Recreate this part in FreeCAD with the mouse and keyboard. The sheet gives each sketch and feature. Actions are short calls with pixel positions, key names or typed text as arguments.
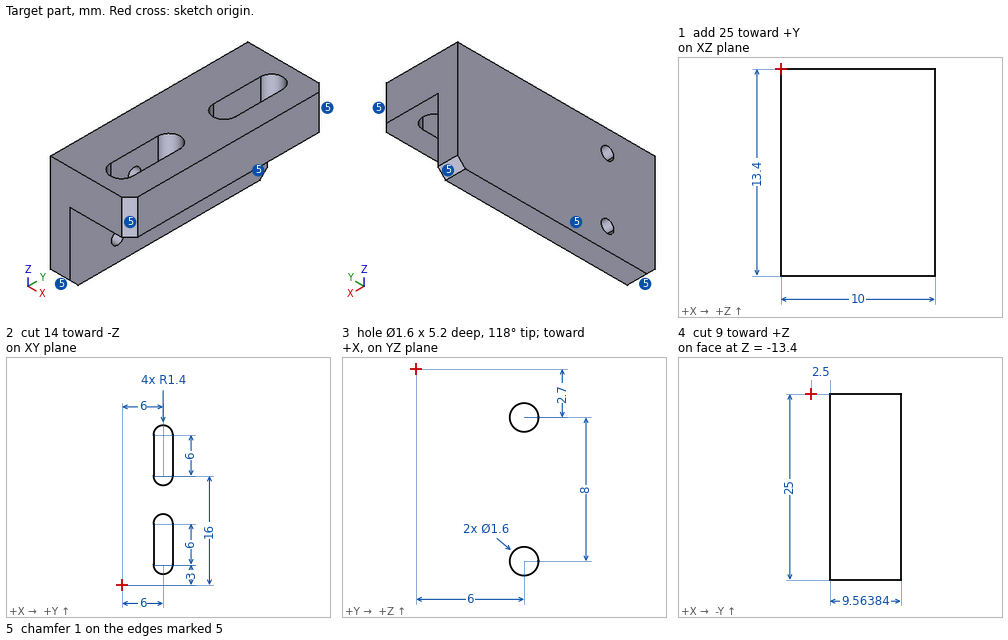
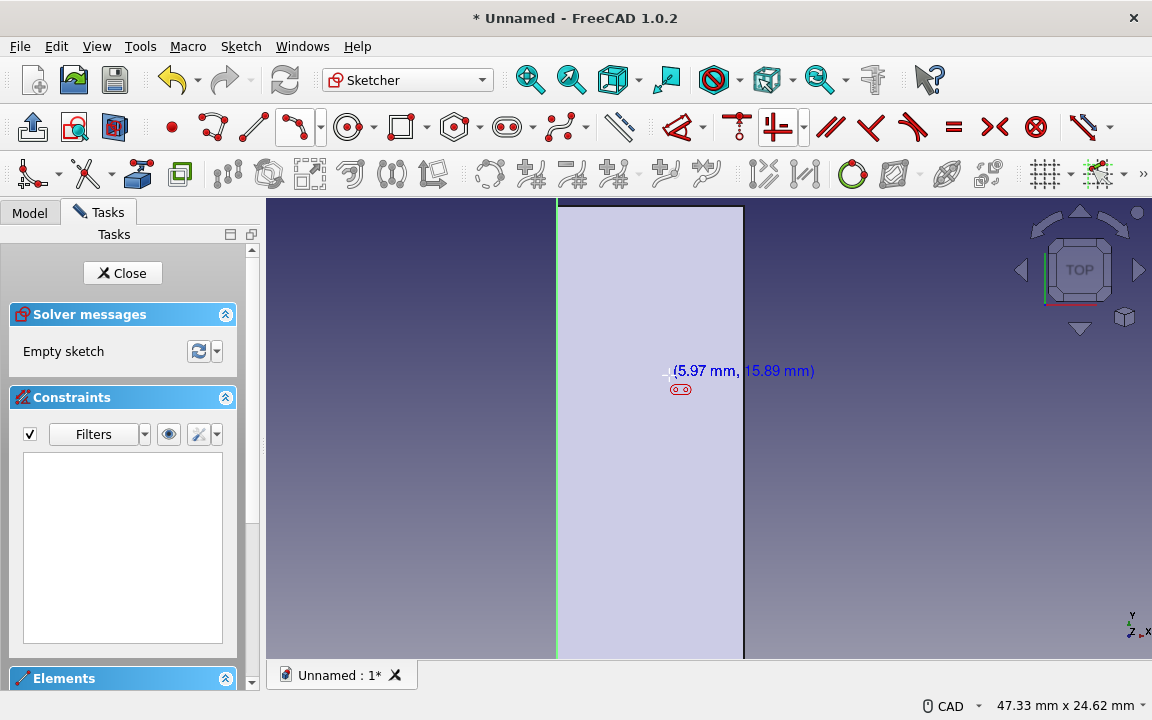
click(669, 374)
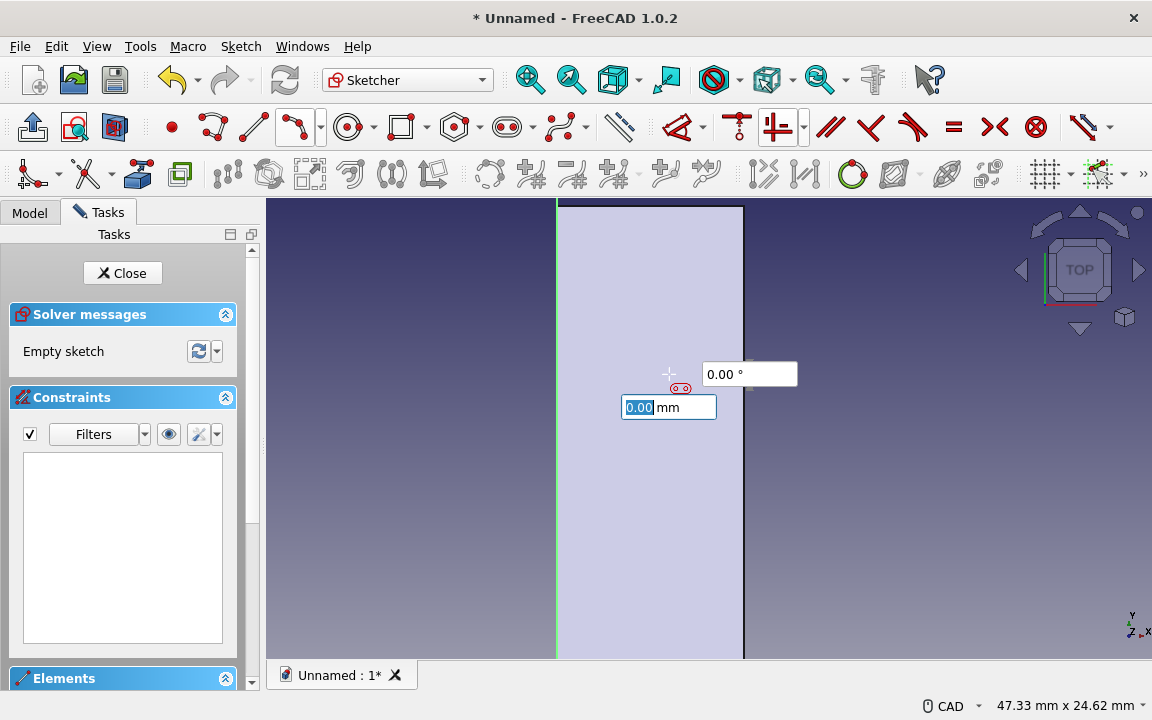
click(669, 262)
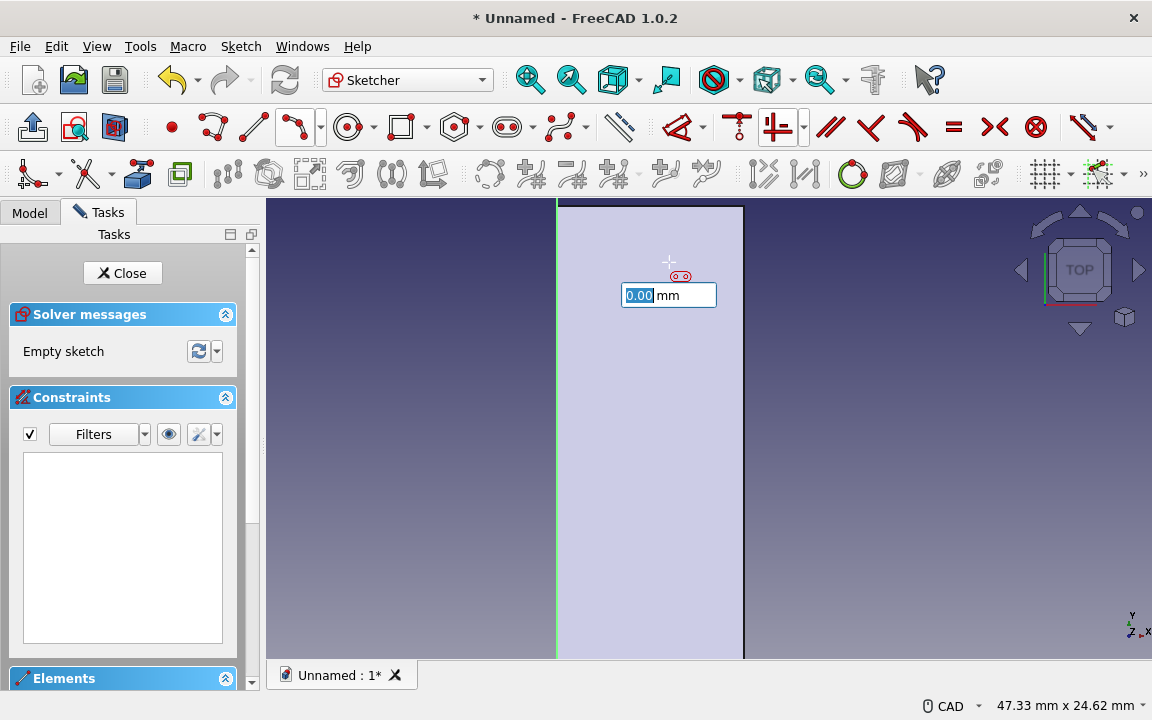
click(696, 318)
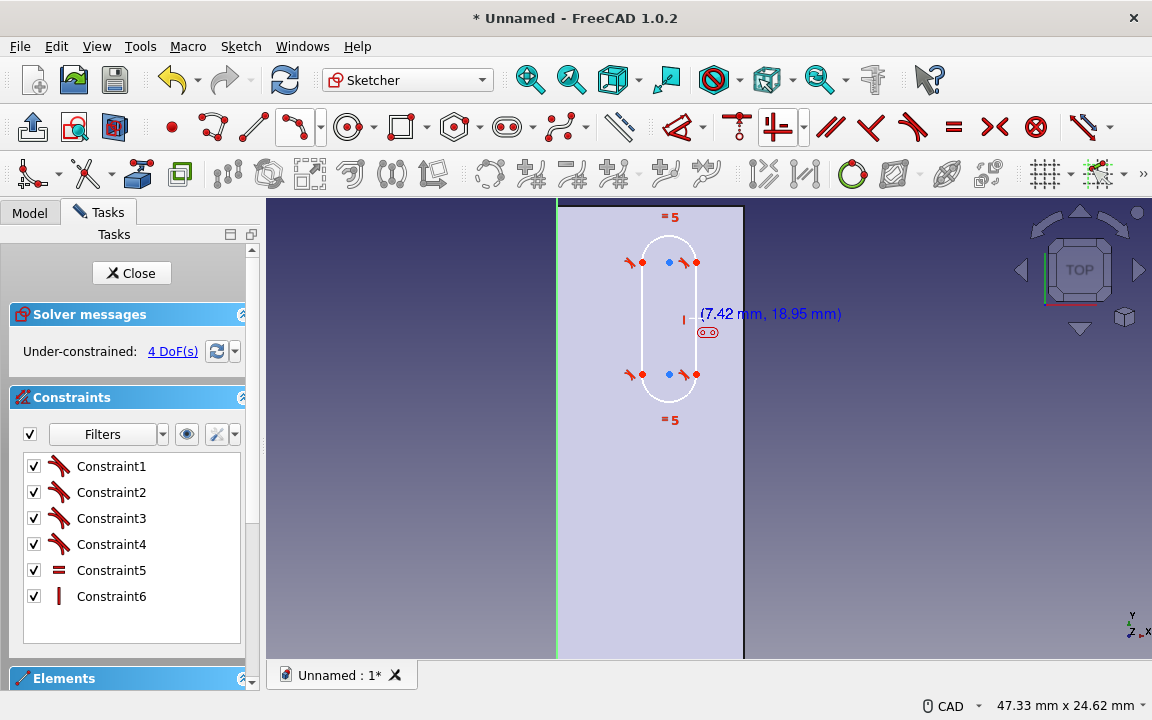
click(669, 618)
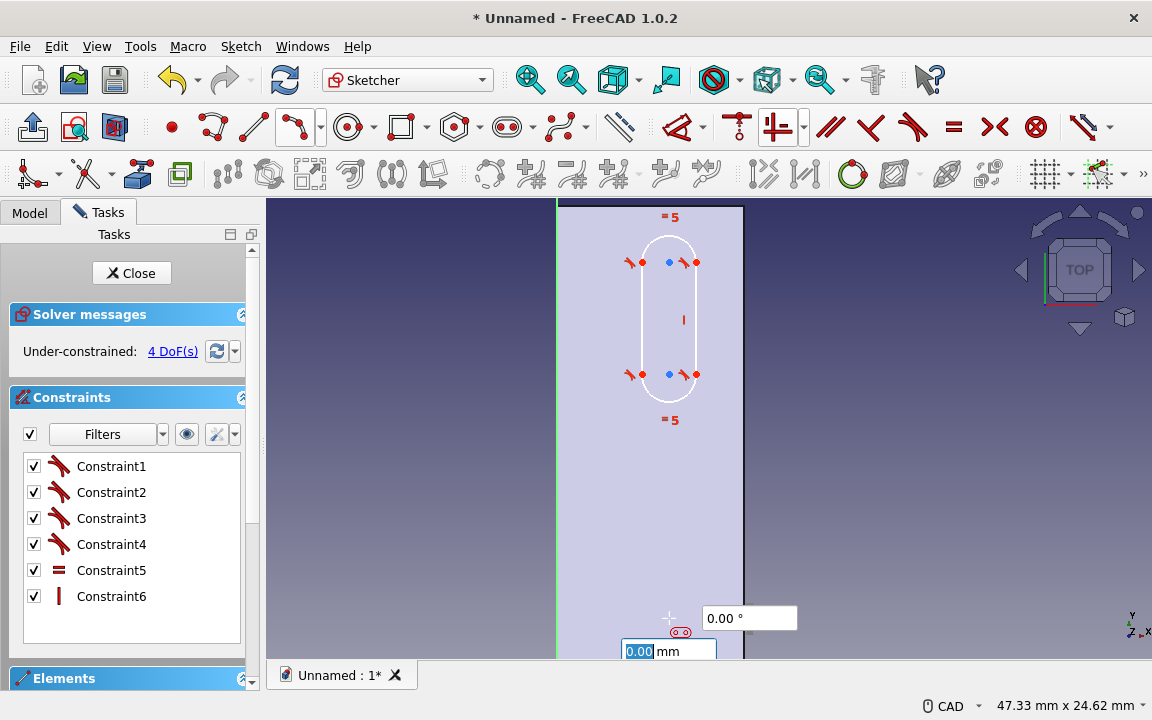
click(669, 505)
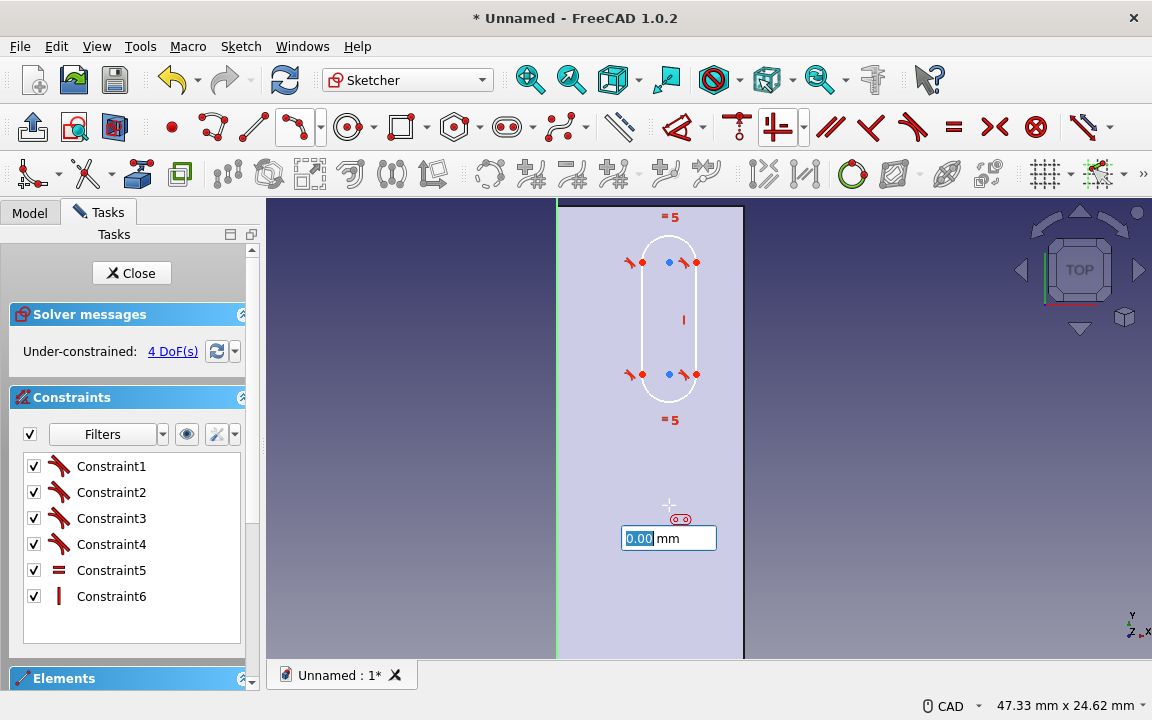
click(696, 561)
key(Escape)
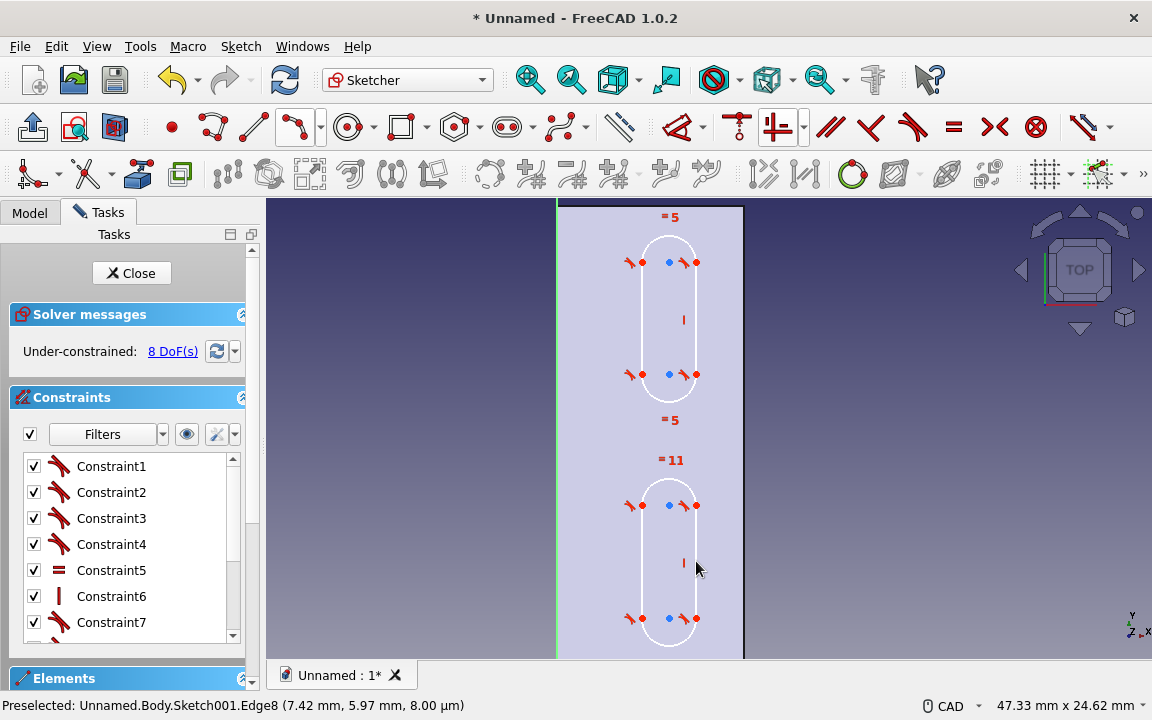
click(653, 397)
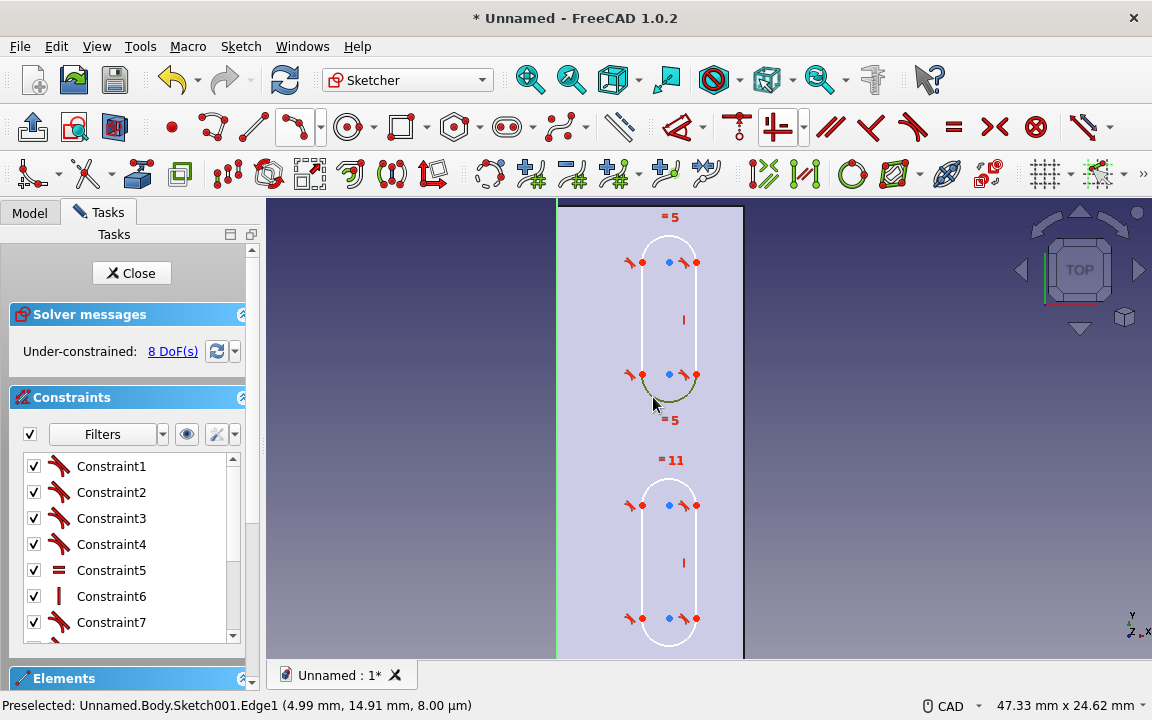
scroll(669, 375, down, 2)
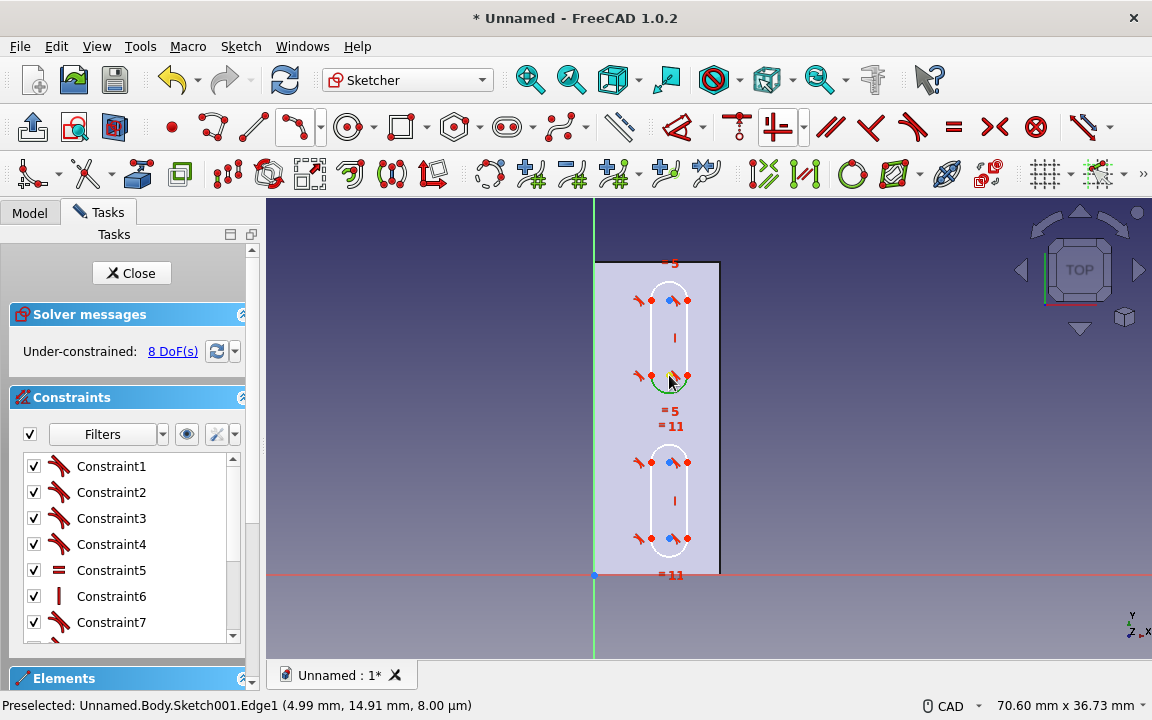
click(659, 553)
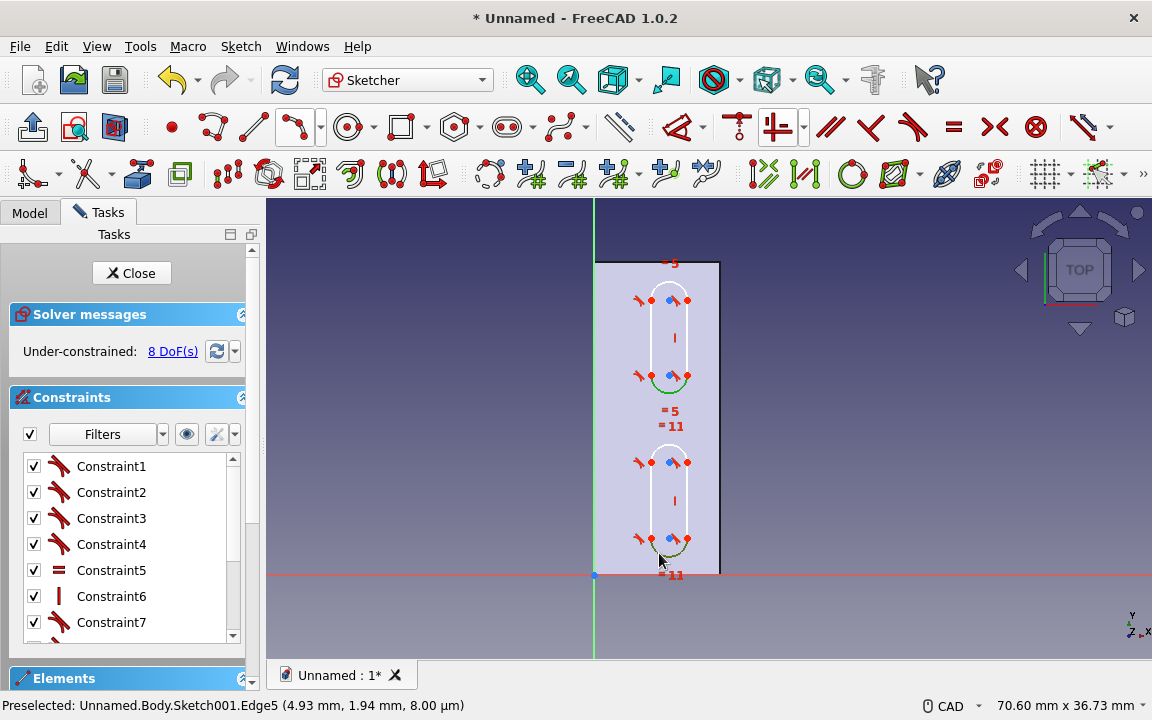
click(954, 128)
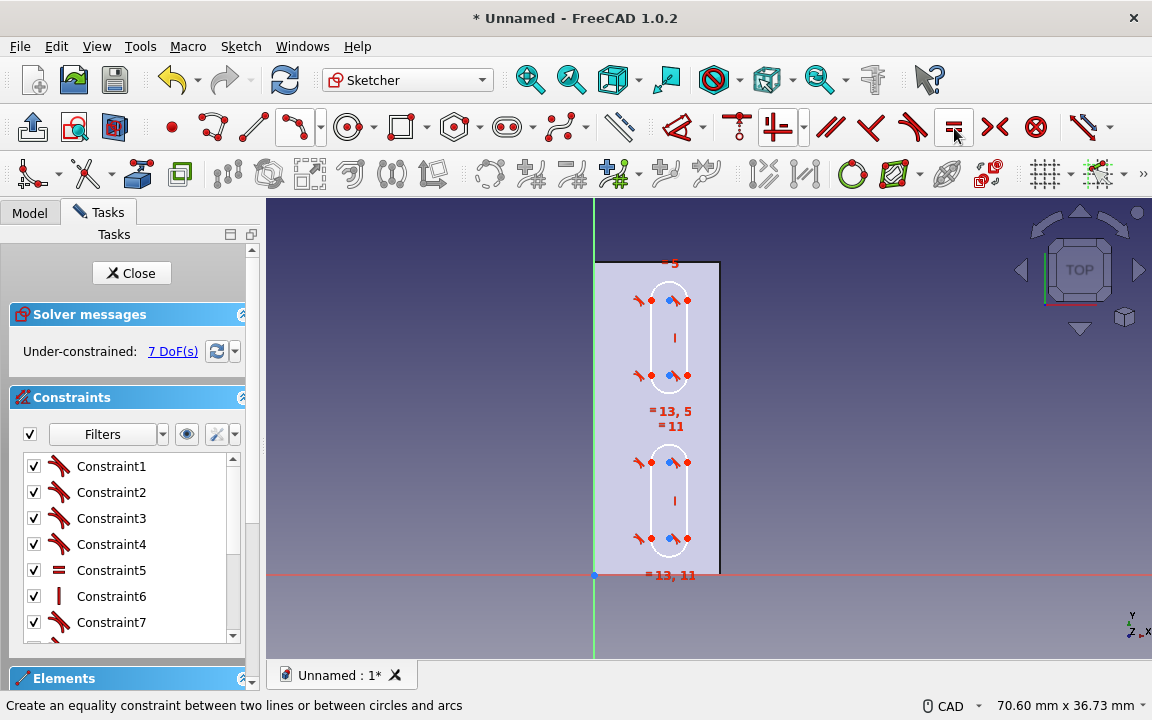
key(d)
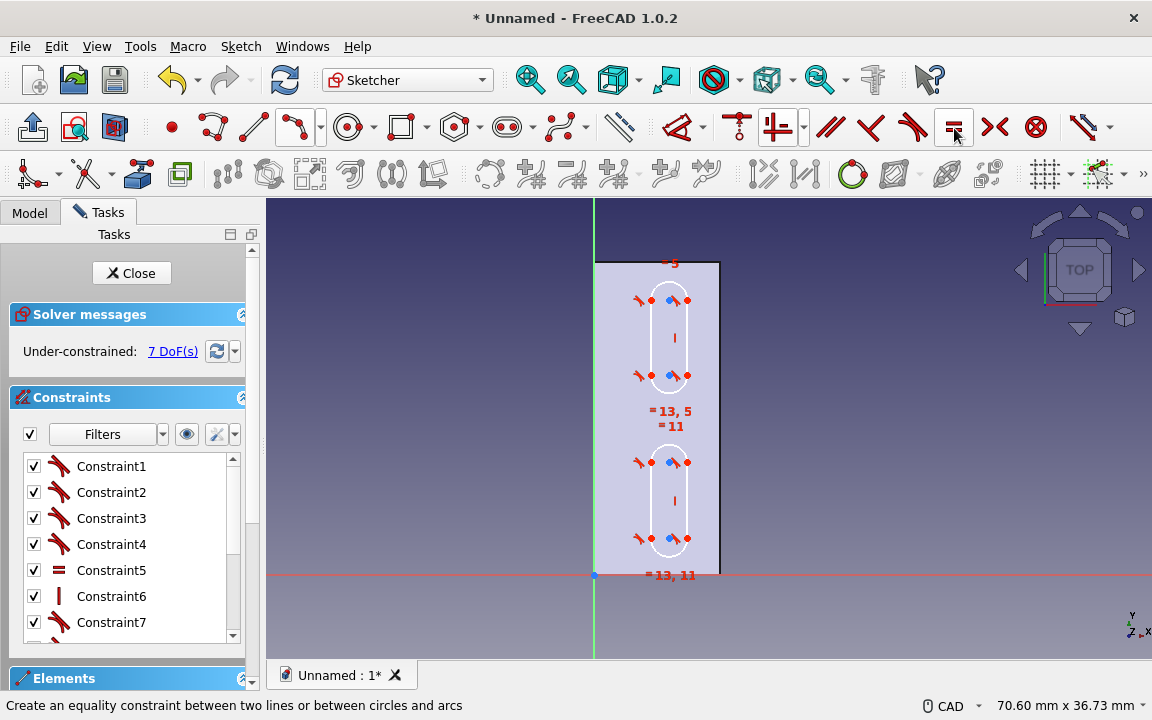
scroll(659, 390, up, 5)